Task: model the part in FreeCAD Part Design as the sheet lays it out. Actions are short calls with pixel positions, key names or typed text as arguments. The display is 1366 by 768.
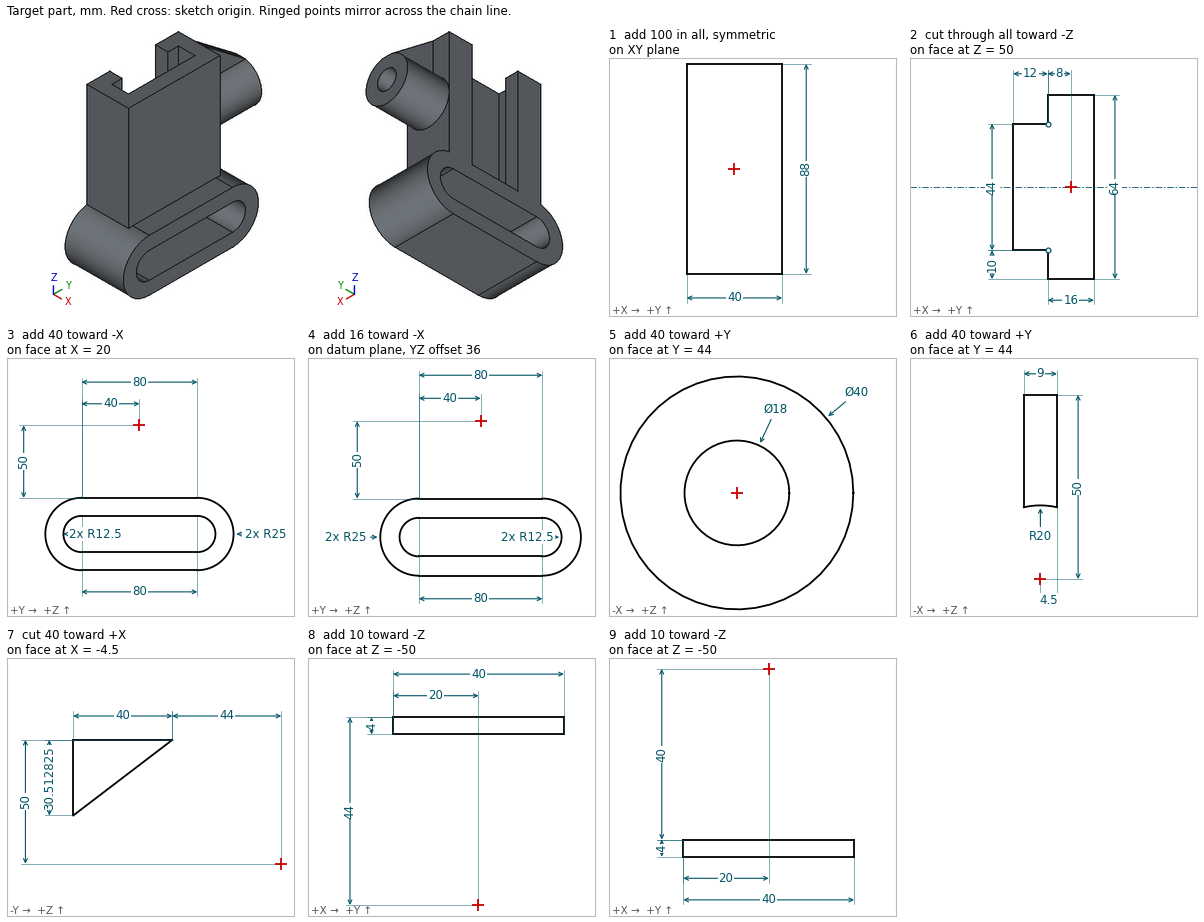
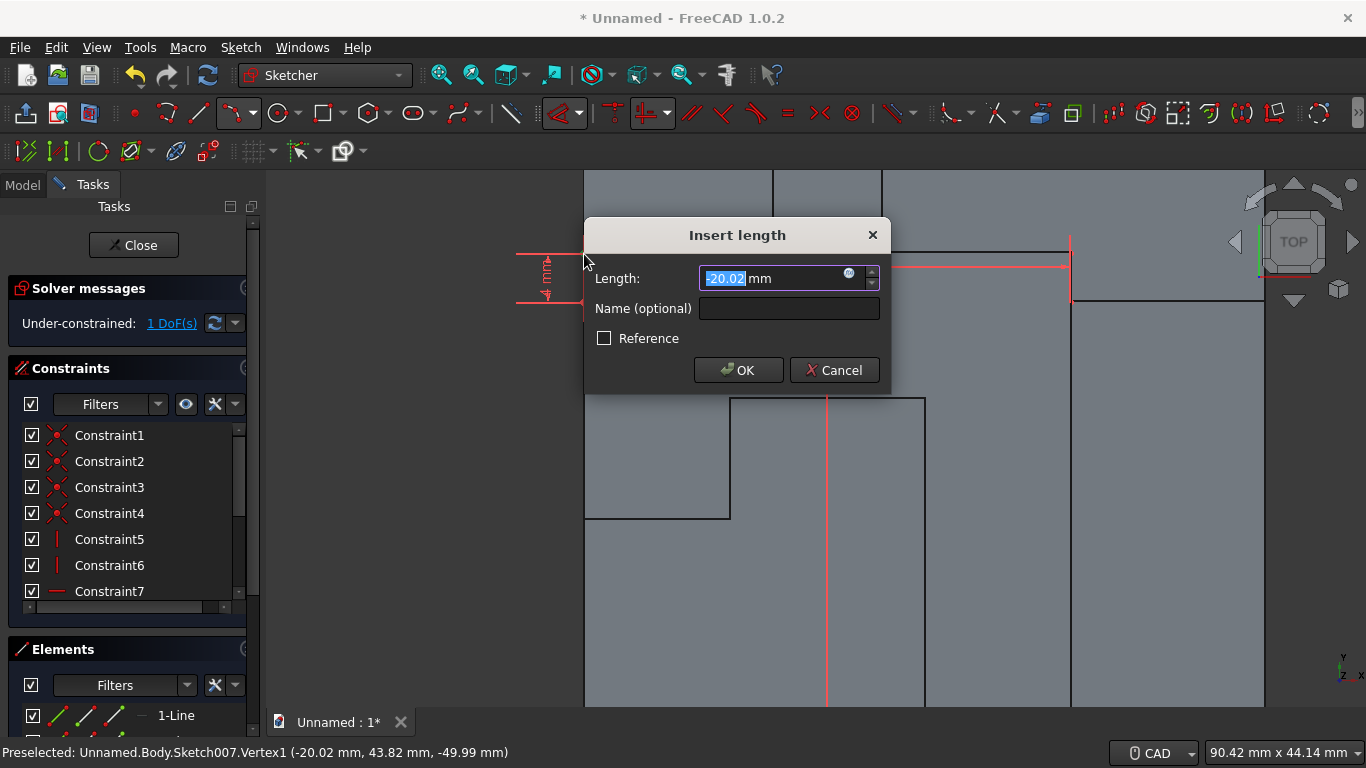
text(-20)
key(Return)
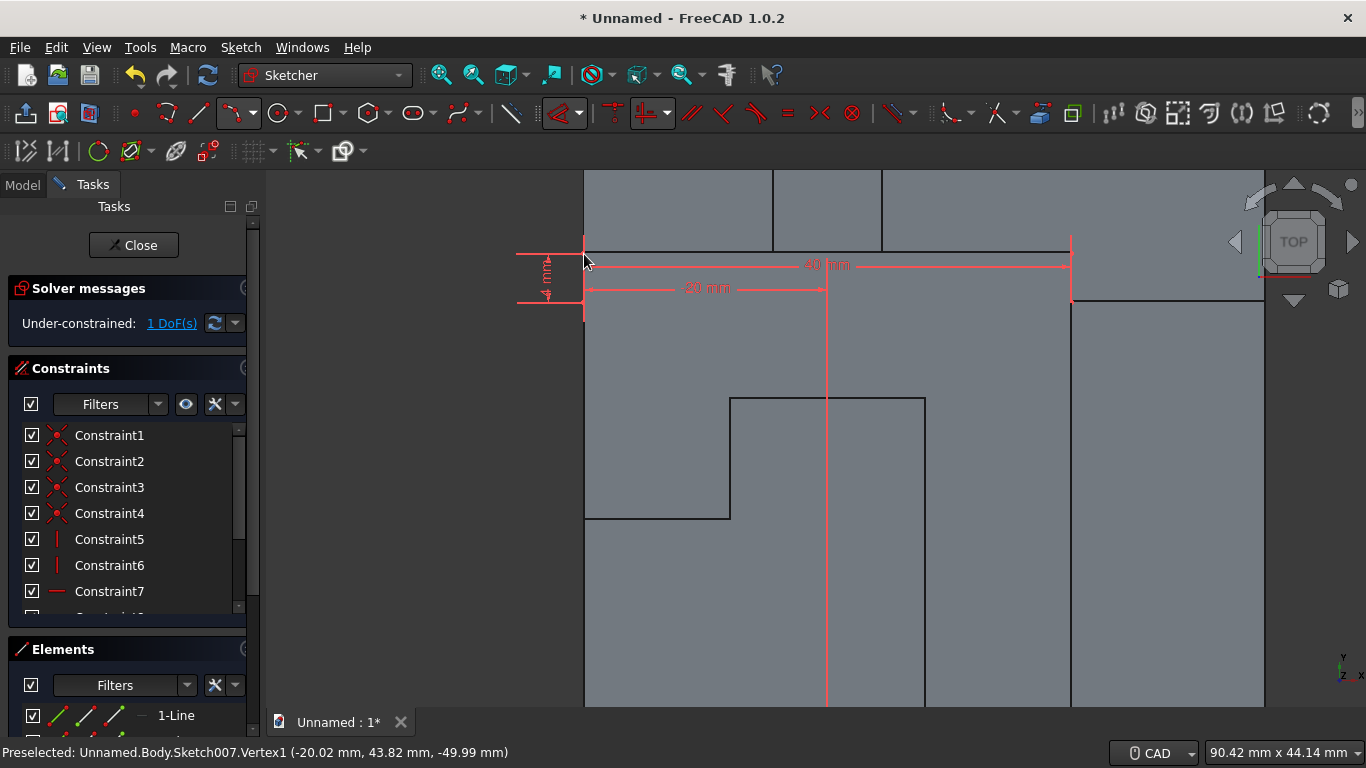
click(584, 254)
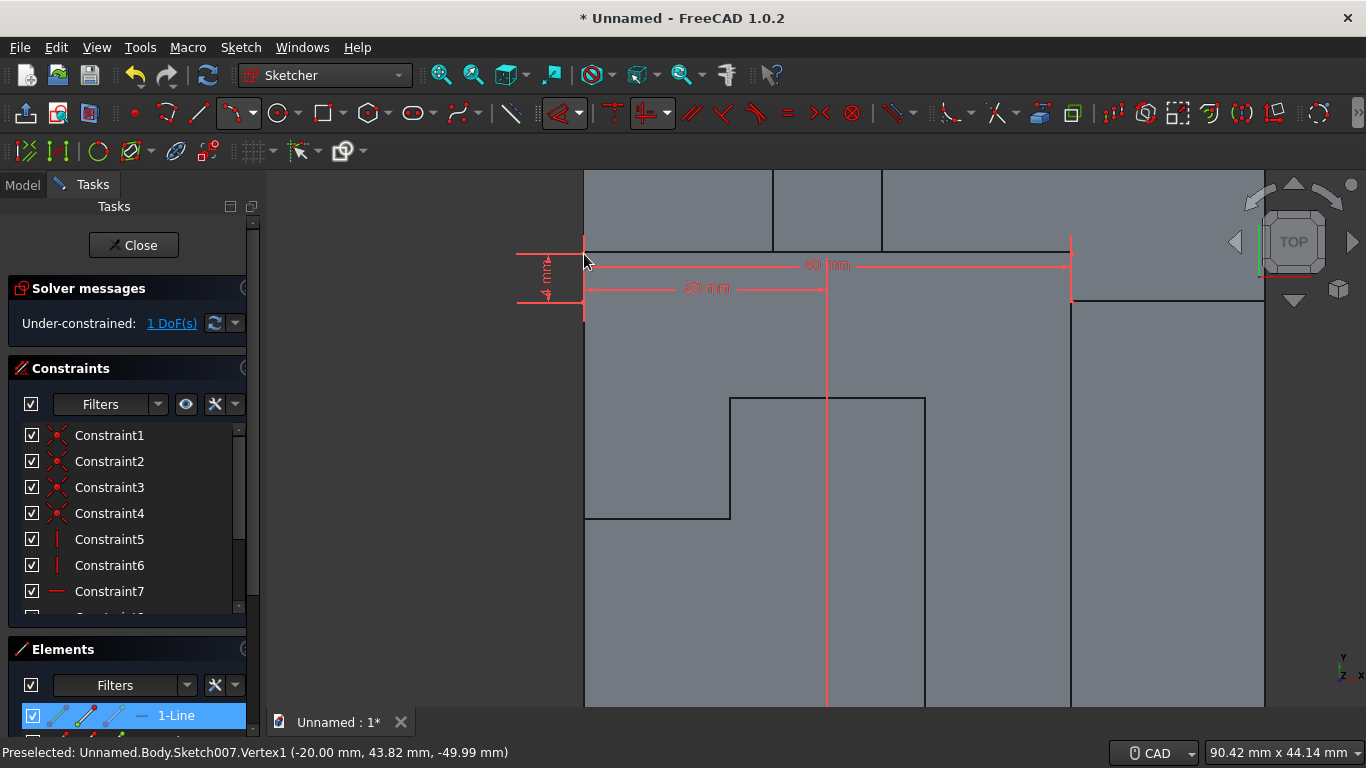
click(582, 114)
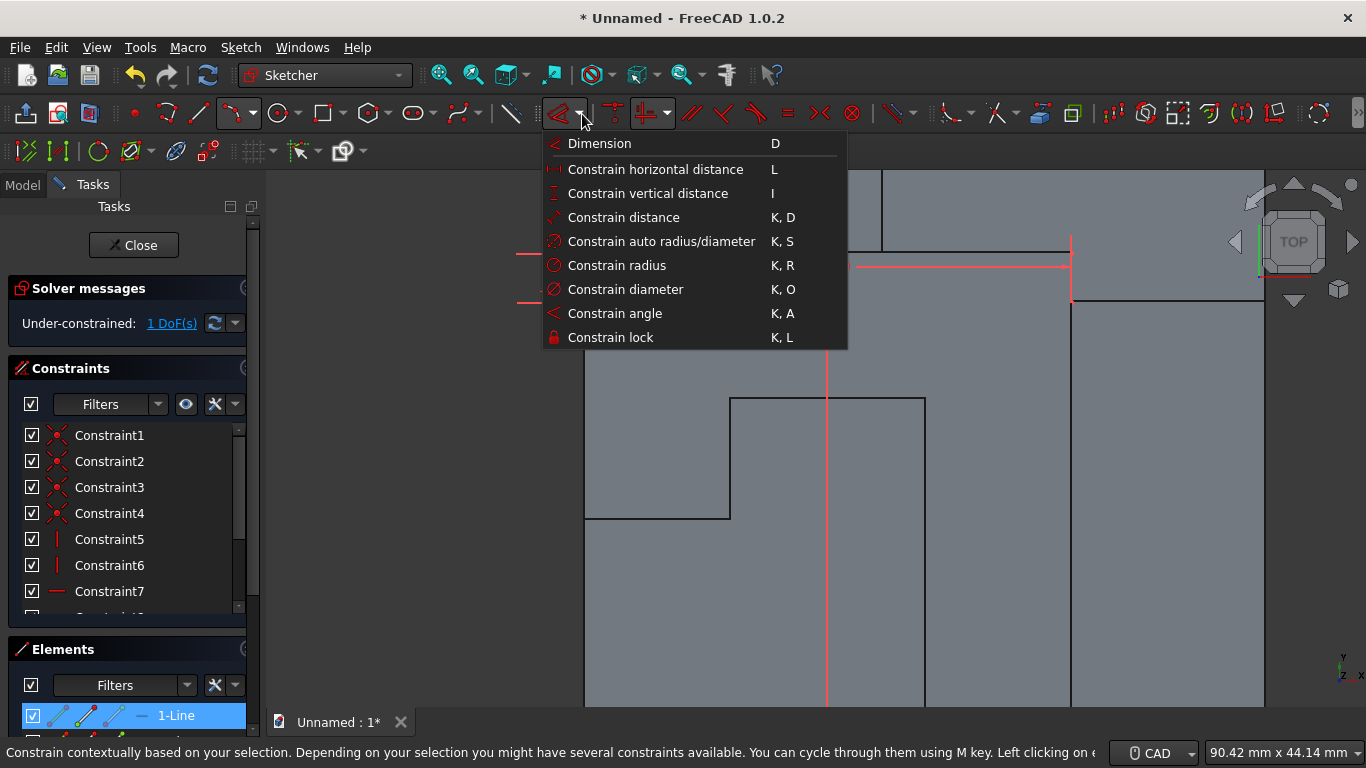
click(695, 193)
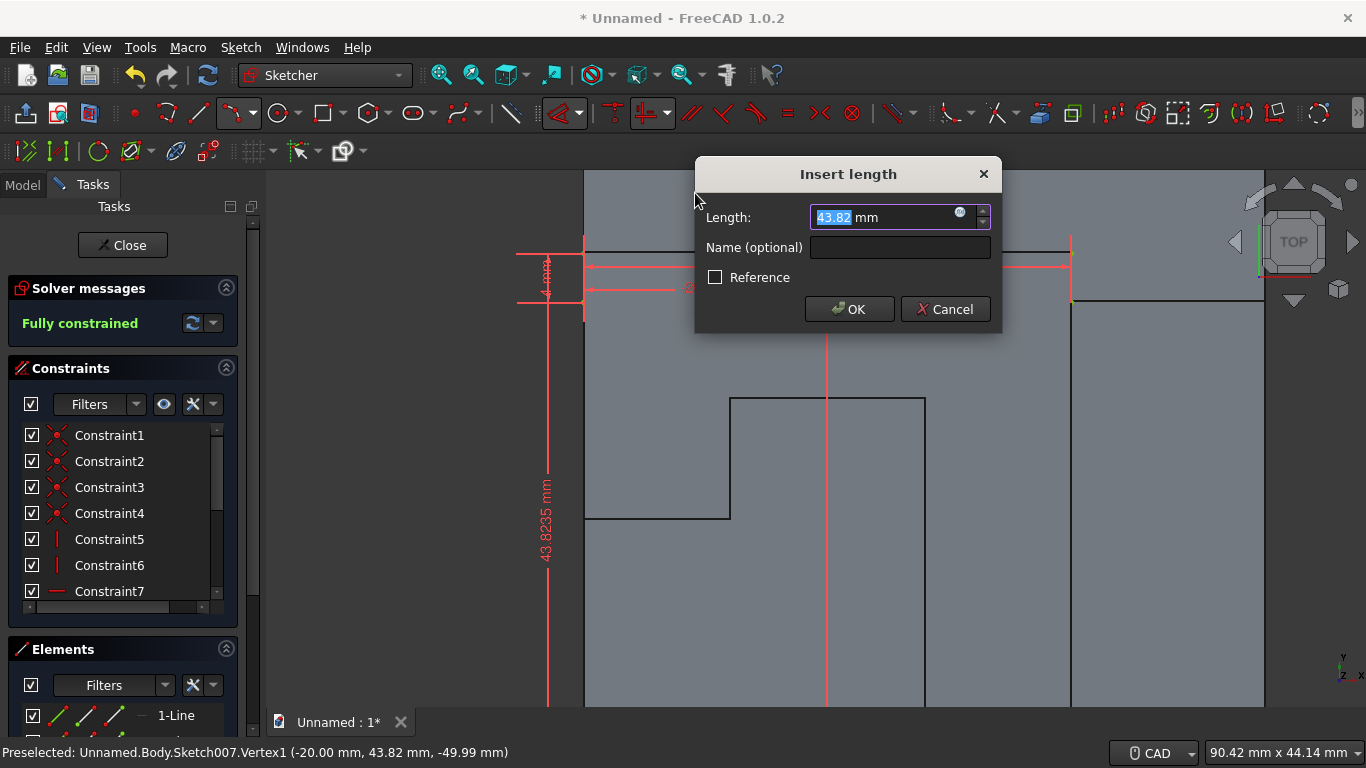
text(44)
key(Return)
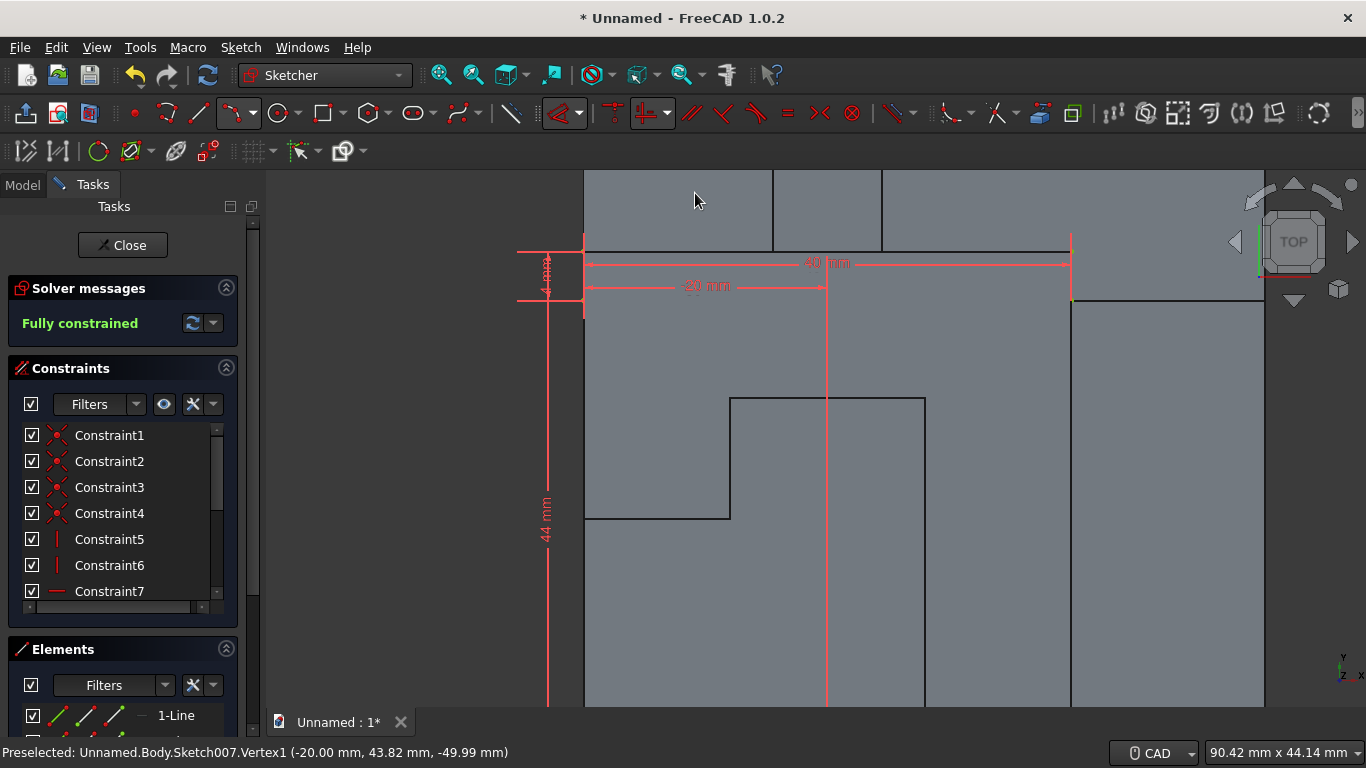
click(123, 245)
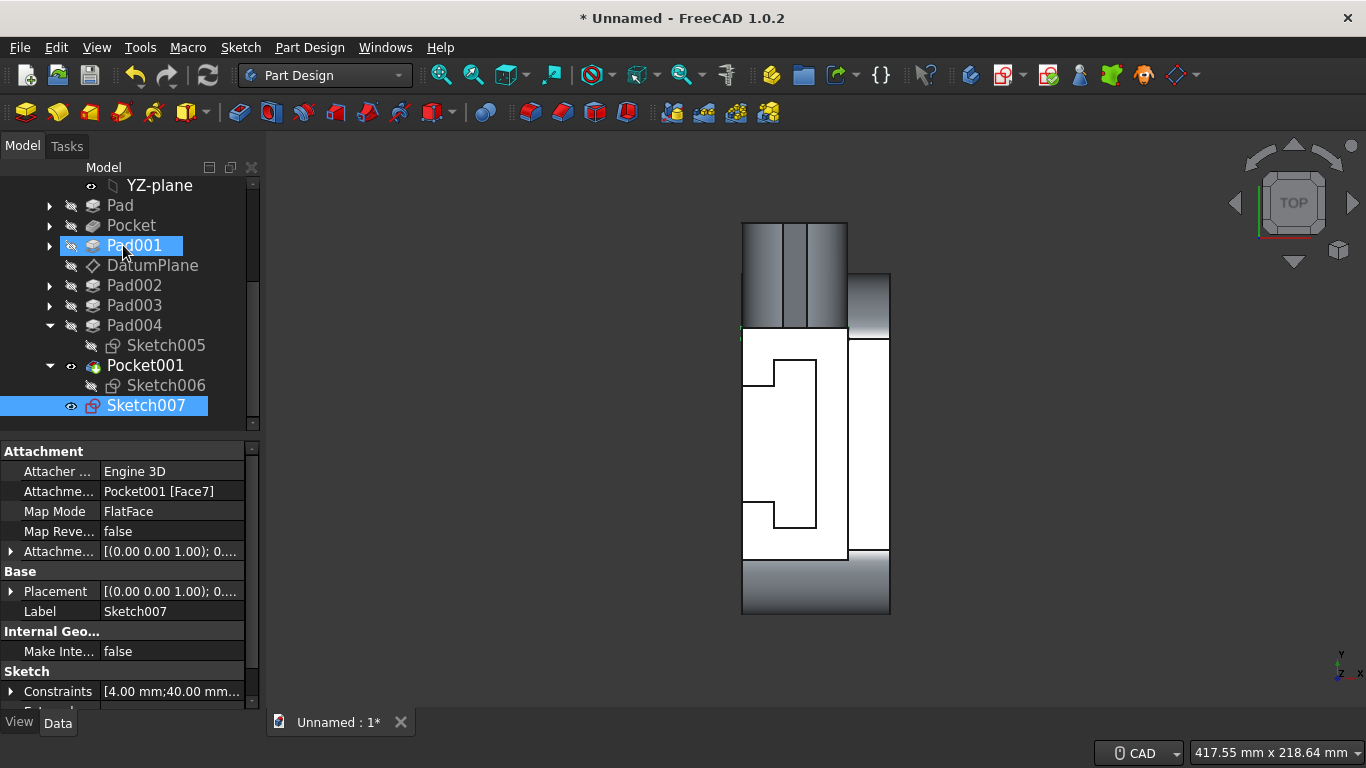
click(26, 112)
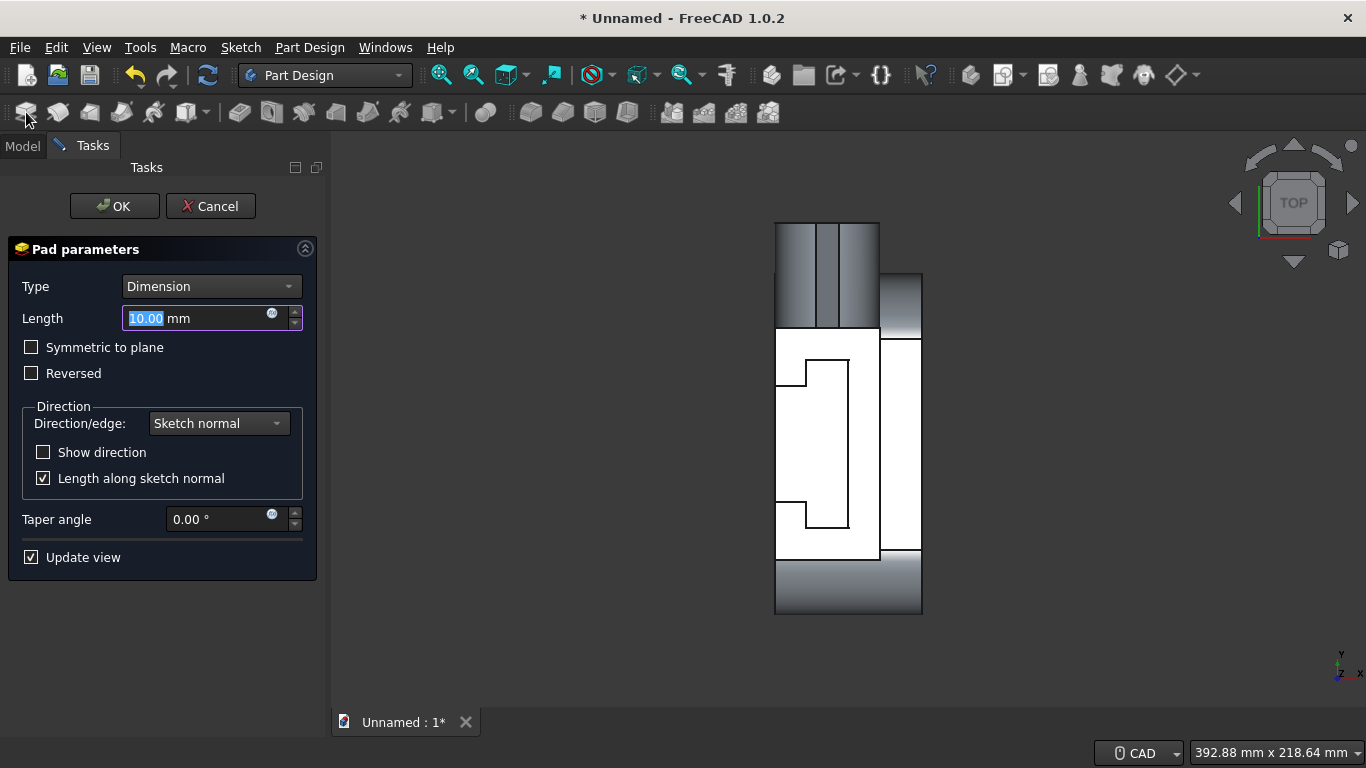
text(10)
key(Tab)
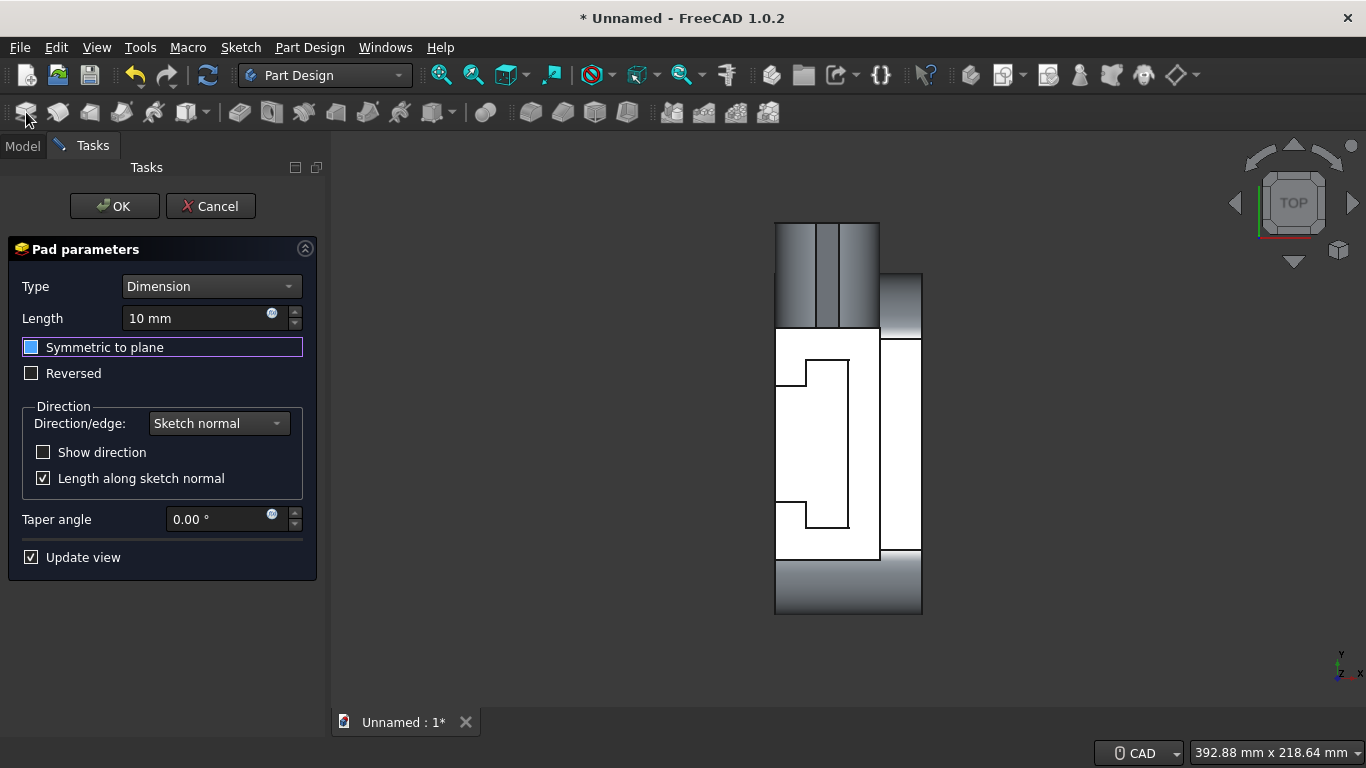
click(30, 373)